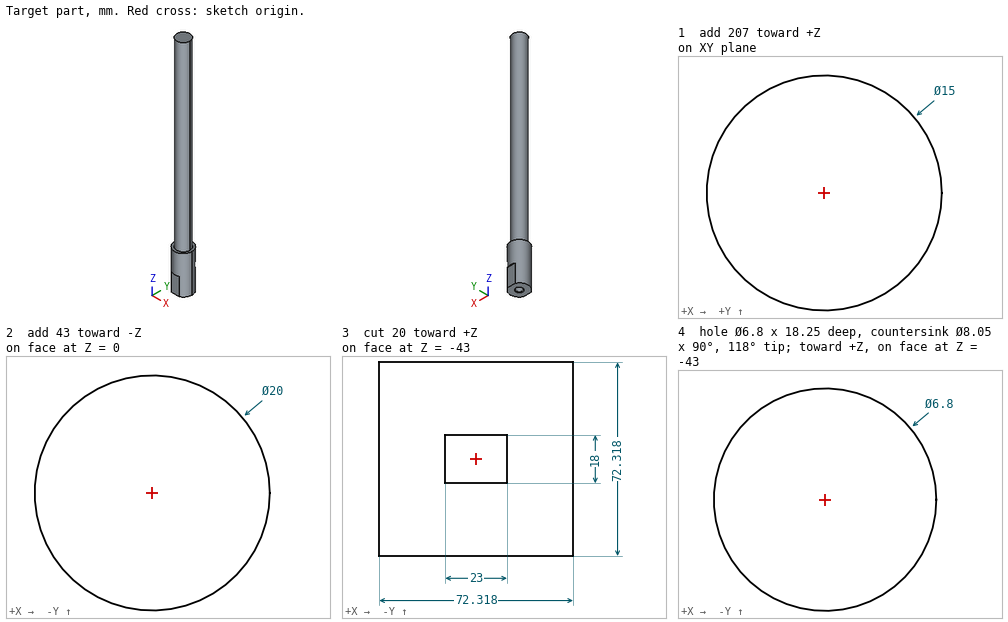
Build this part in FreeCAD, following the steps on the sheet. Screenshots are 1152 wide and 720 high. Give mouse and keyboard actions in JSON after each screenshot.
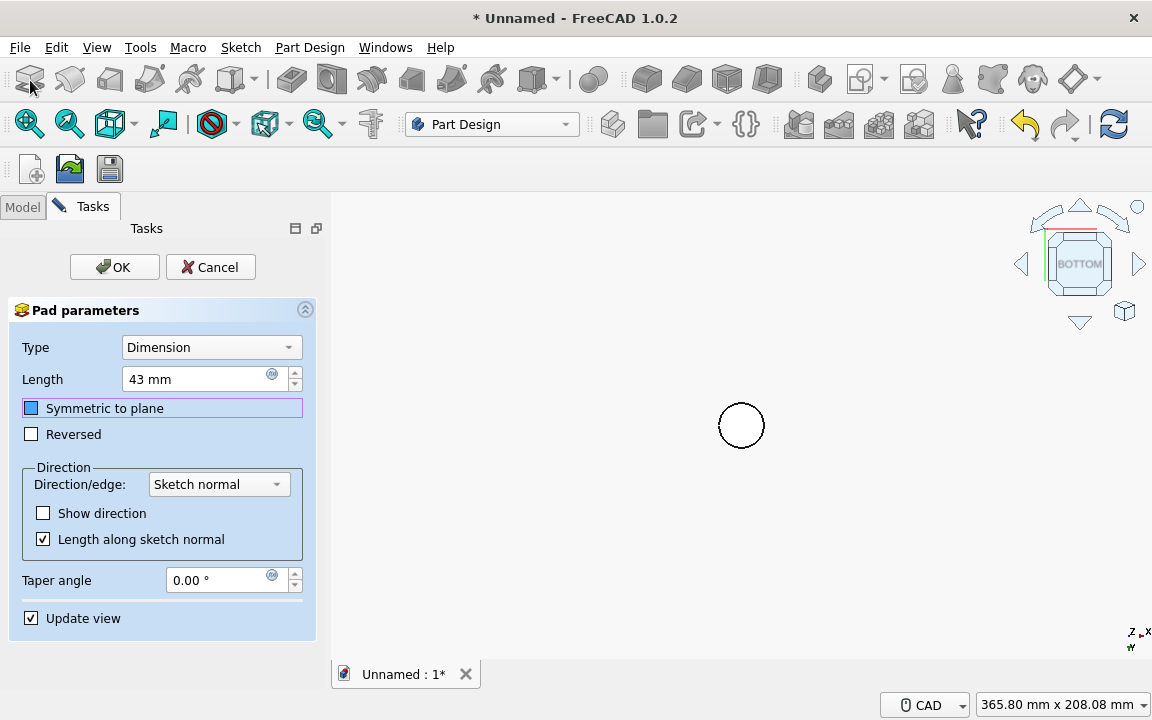
{"action": "left_click", "coordinate": [115, 267]}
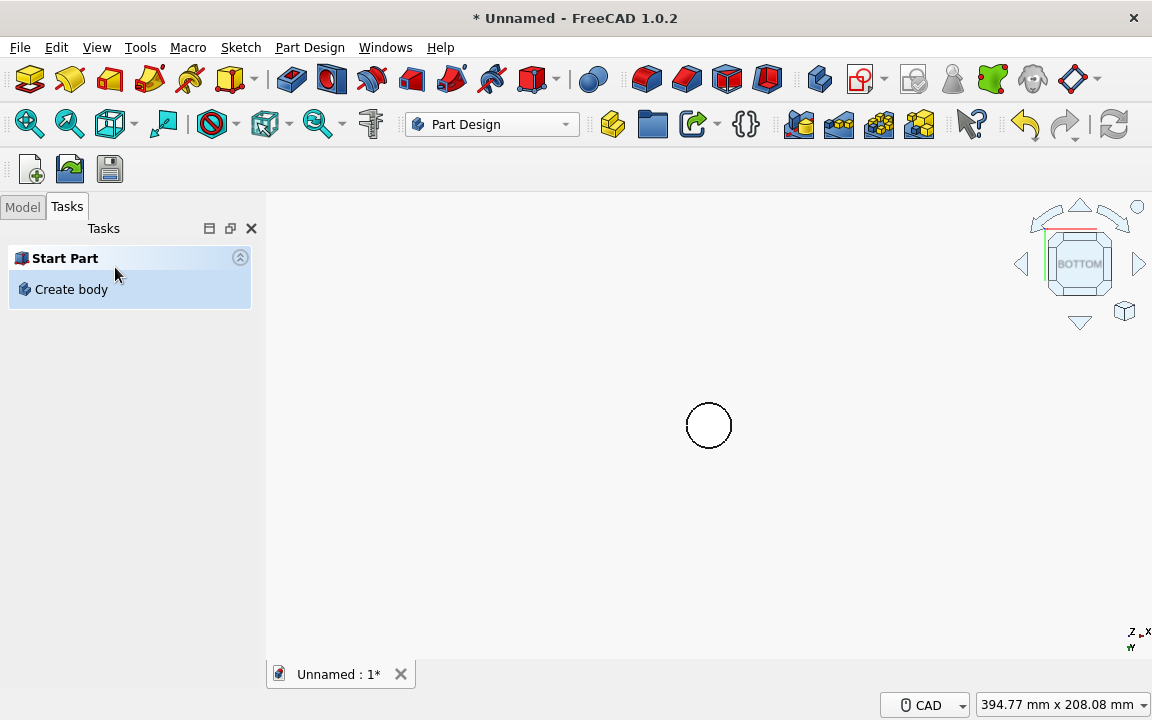
{"action": "key", "text": "v f"}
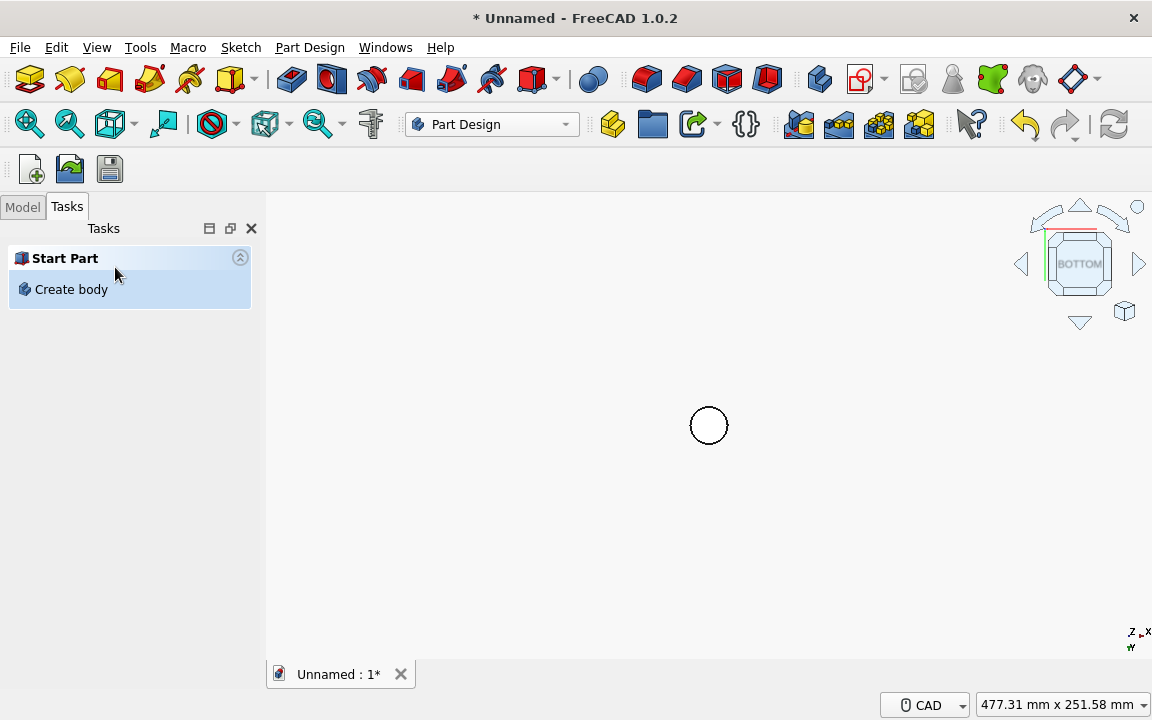
{"action": "left_click", "coordinate": [709, 424]}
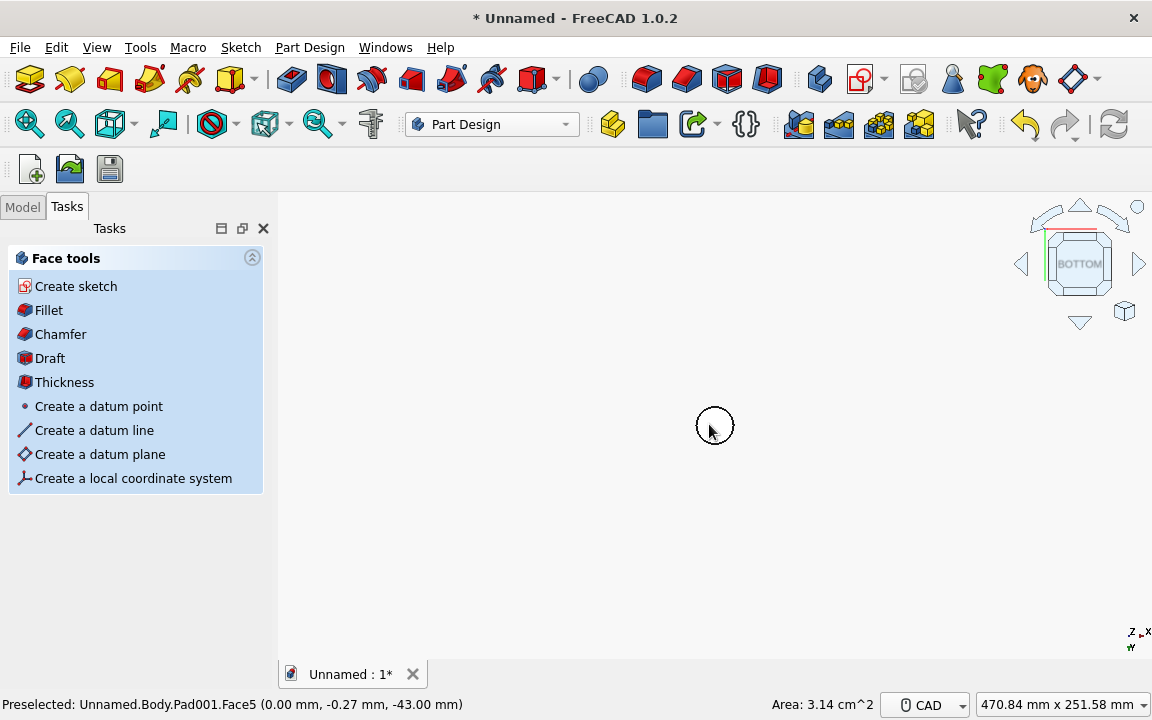
{"action": "left_click", "coordinate": [860, 80]}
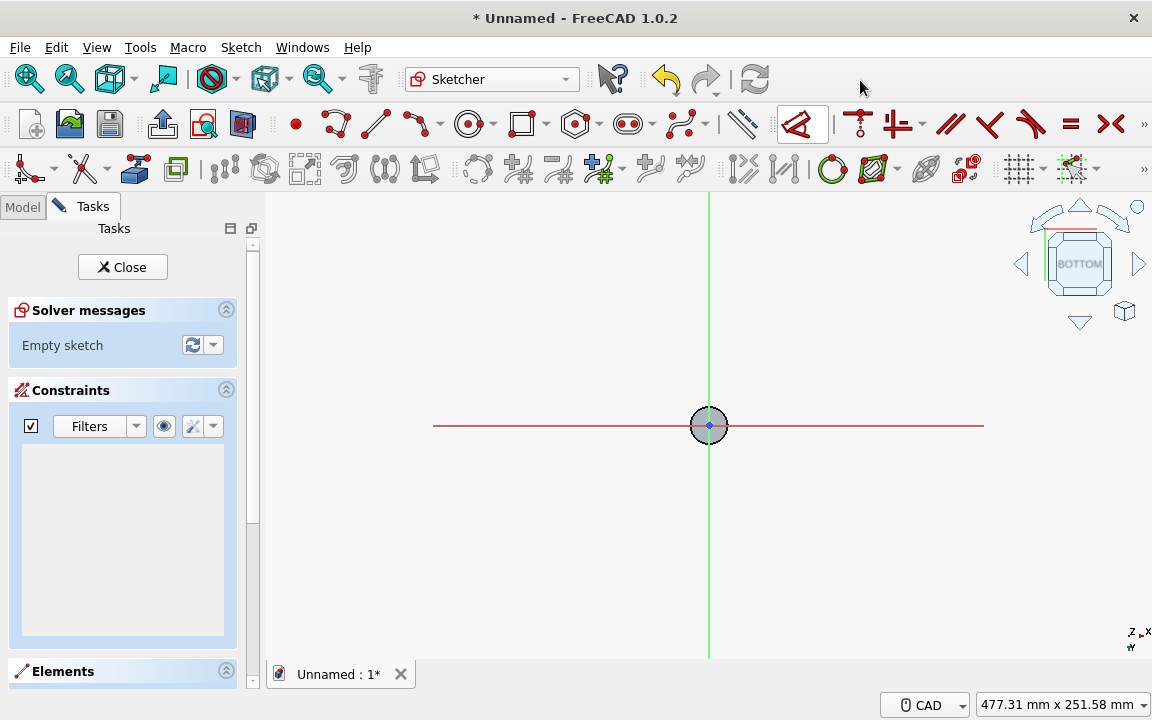
{"action": "scroll", "coordinate": [765, 426], "scroll_direction": "up", "scroll_amount": 4}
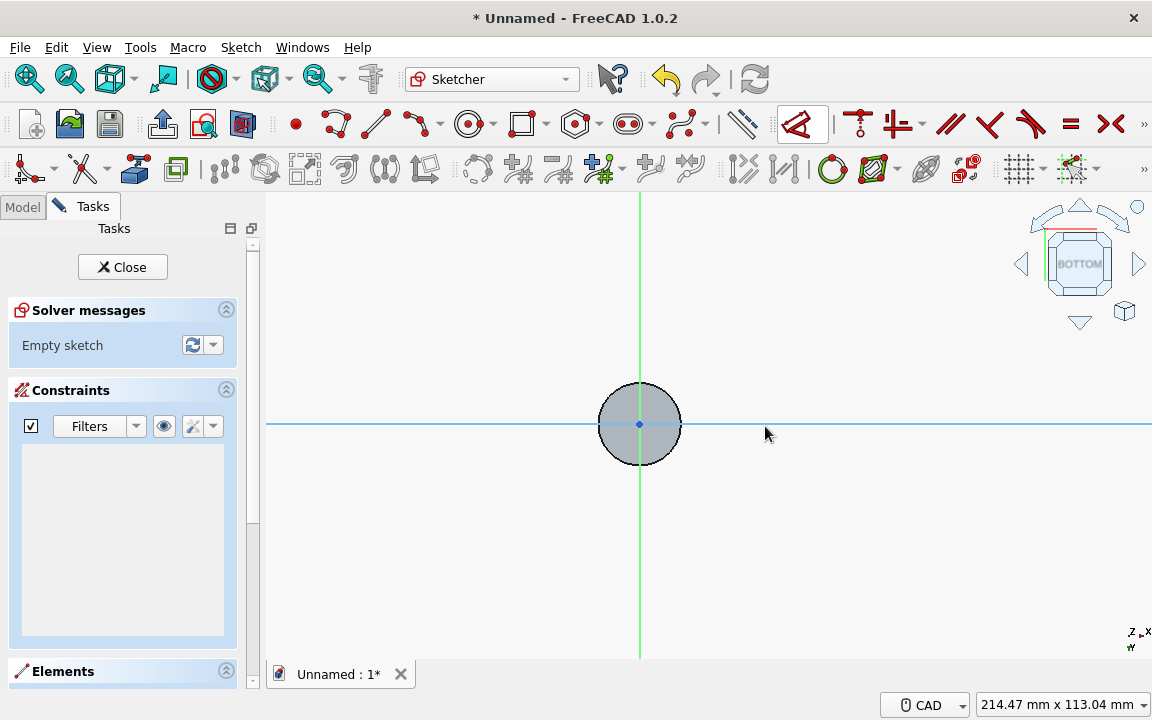
{"action": "left_click", "coordinate": [548, 124]}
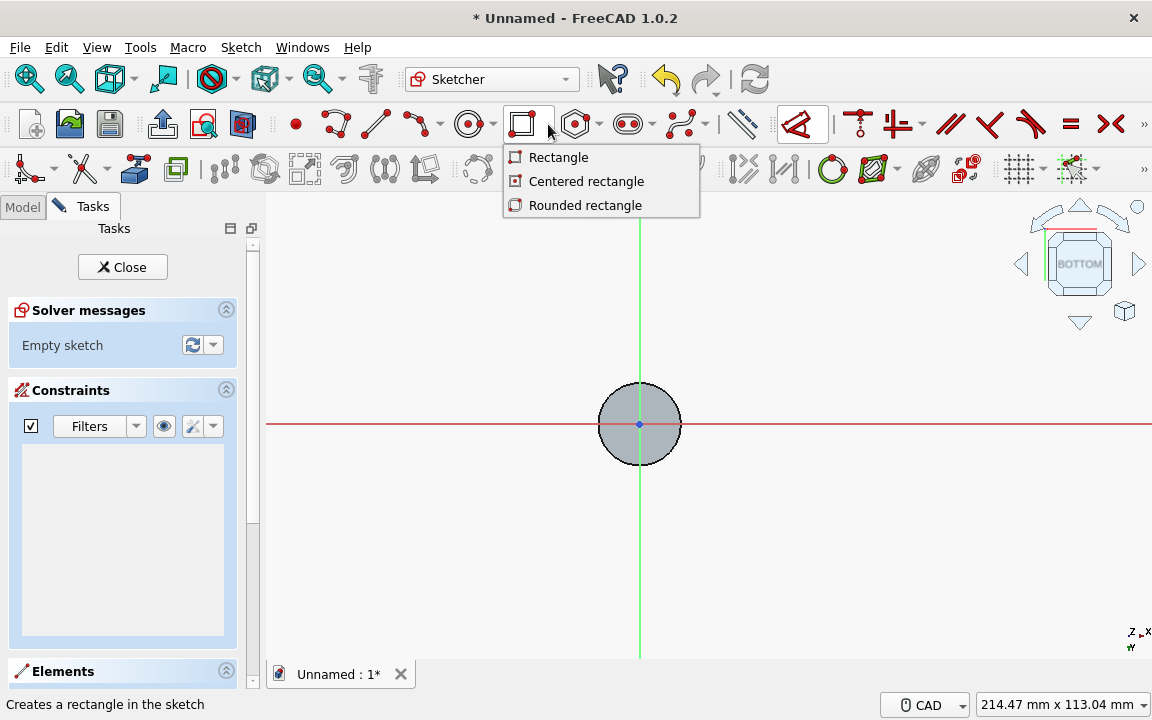
{"action": "left_click", "coordinate": [602, 181]}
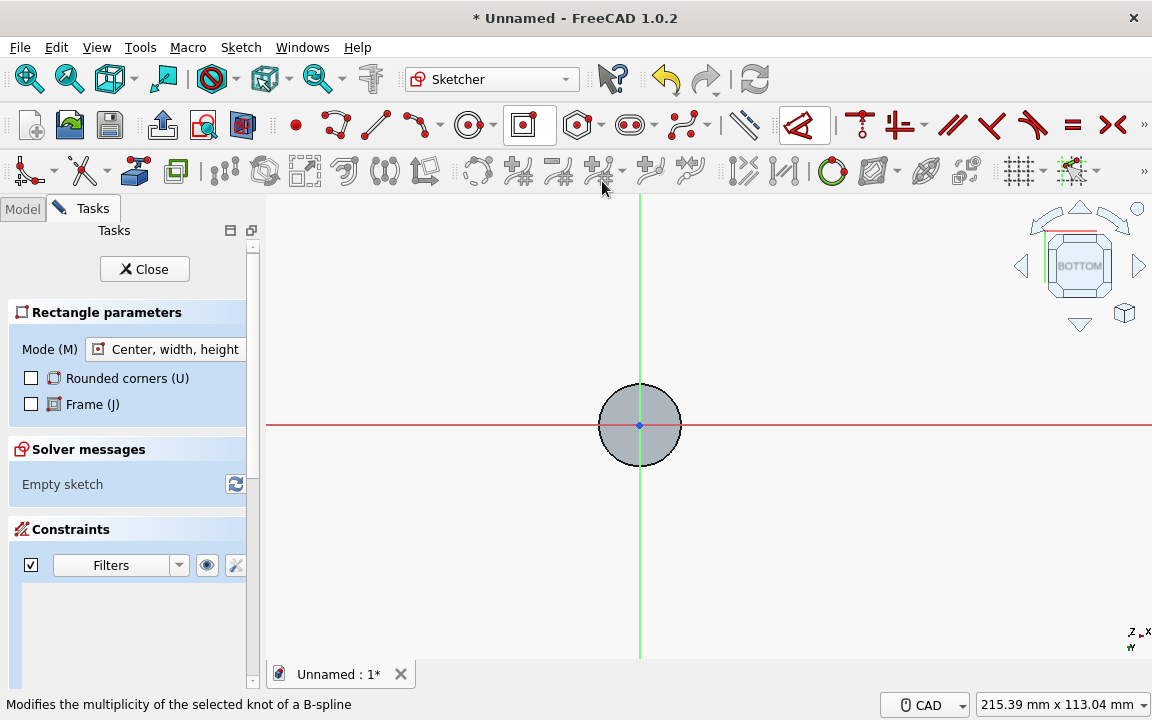
{"action": "left_click", "coordinate": [640, 425]}
{"action": "mouse_move", "coordinate": [789, 277]}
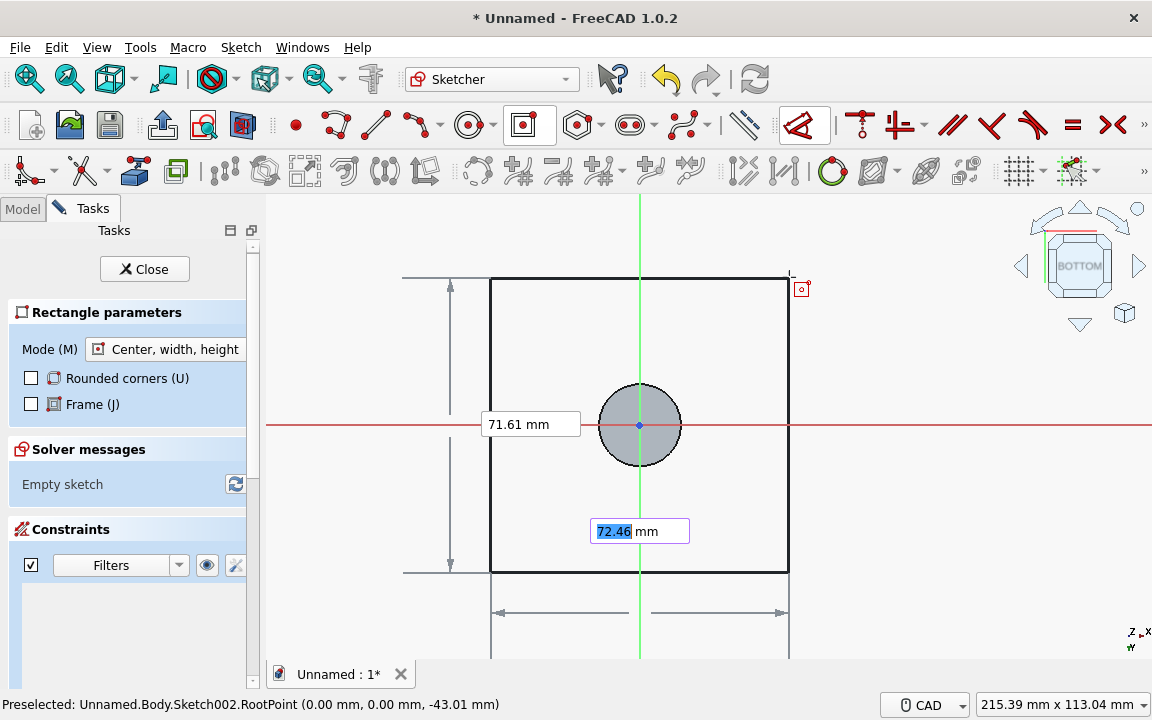
{"action": "type", "text": "72.318"}
{"action": "key", "text": "Tab"}
{"action": "type", "text": "72.318"}
{"action": "key", "text": "Return"}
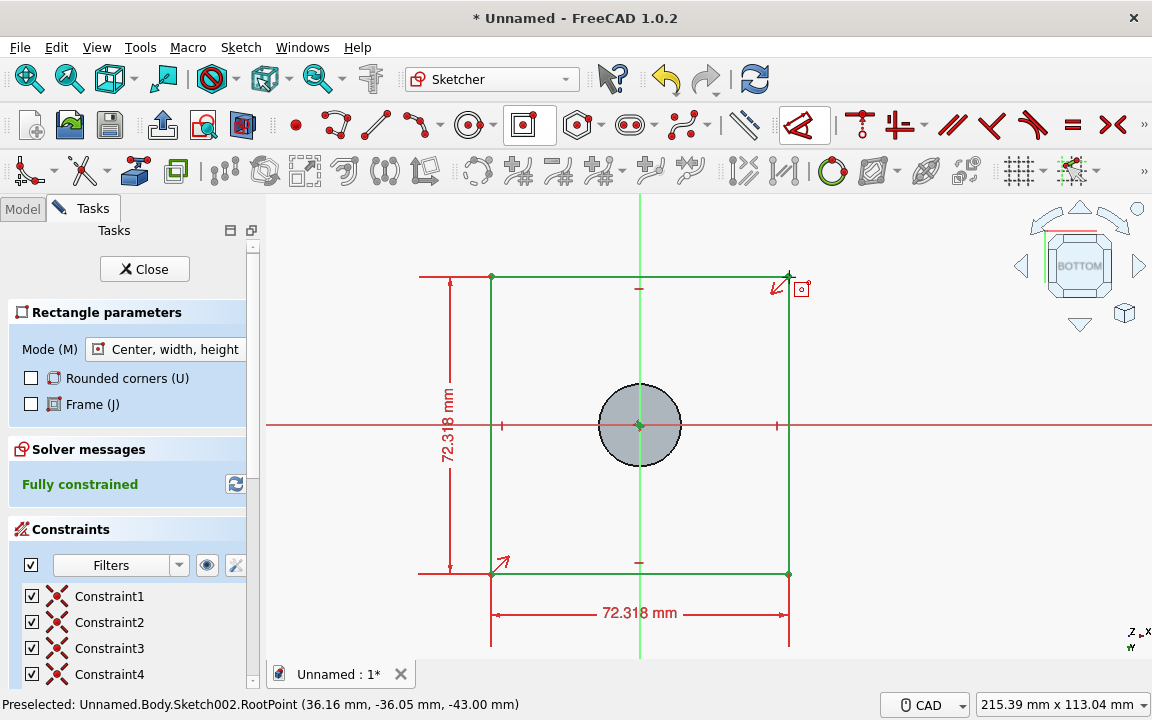
{"action": "left_click", "coordinate": [640, 425]}
{"action": "mouse_move", "coordinate": [687, 388]}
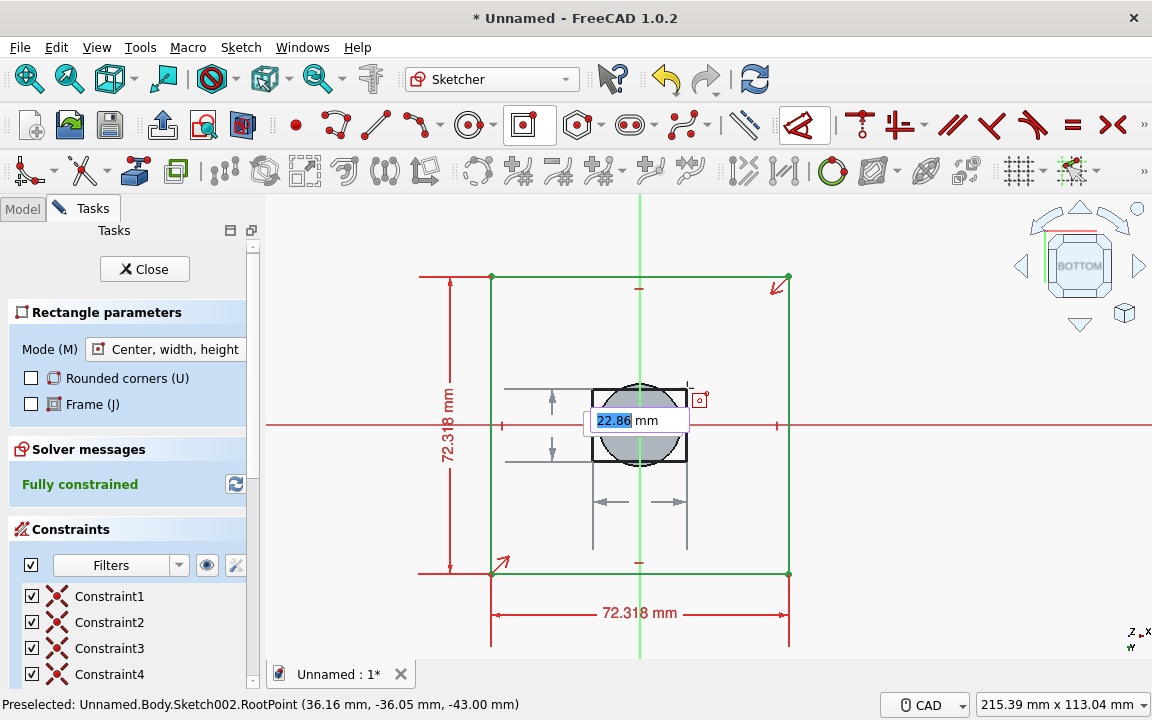
{"action": "type", "text": "23"}
{"action": "key", "text": "Tab"}
{"action": "type", "text": "18"}
{"action": "key", "text": "Return"}
{"action": "key", "text": "Escape"}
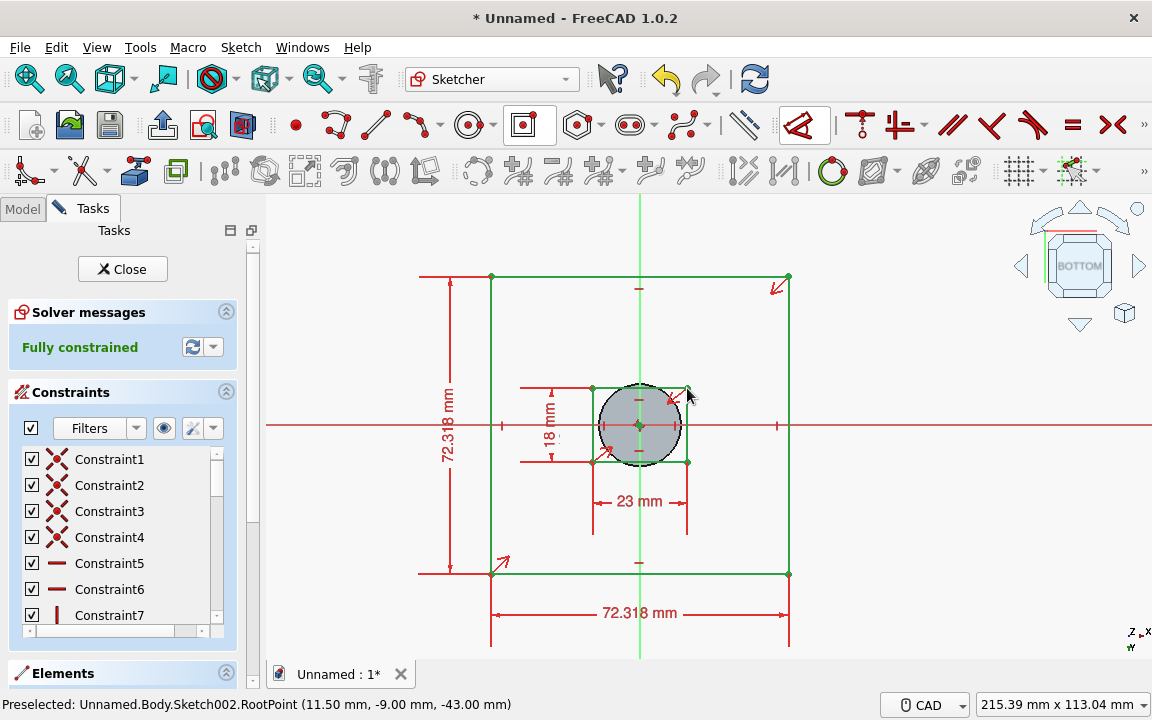
{"action": "left_click", "coordinate": [123, 269]}